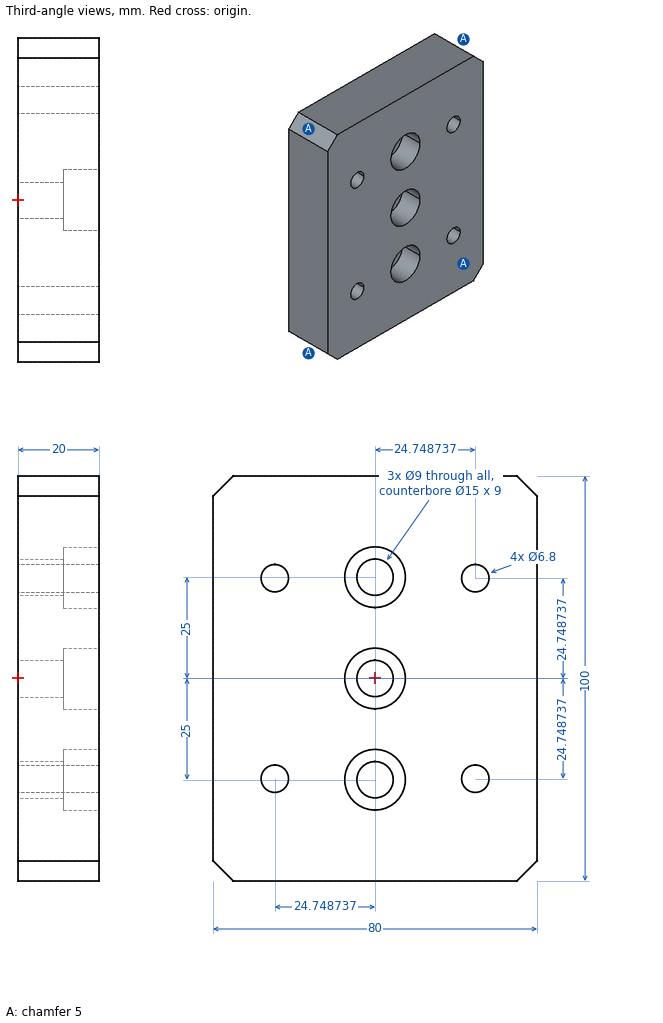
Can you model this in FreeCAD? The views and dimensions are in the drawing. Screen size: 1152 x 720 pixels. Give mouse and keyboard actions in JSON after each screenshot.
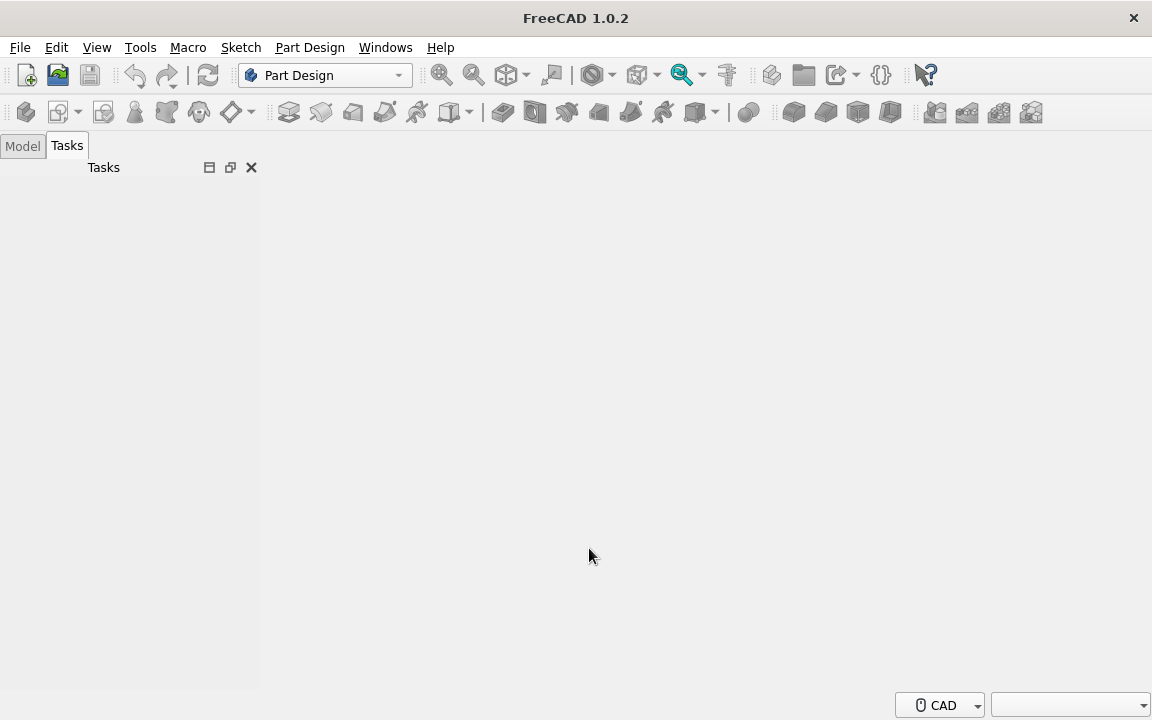
{"action": "key", "text": "ctrl+n"}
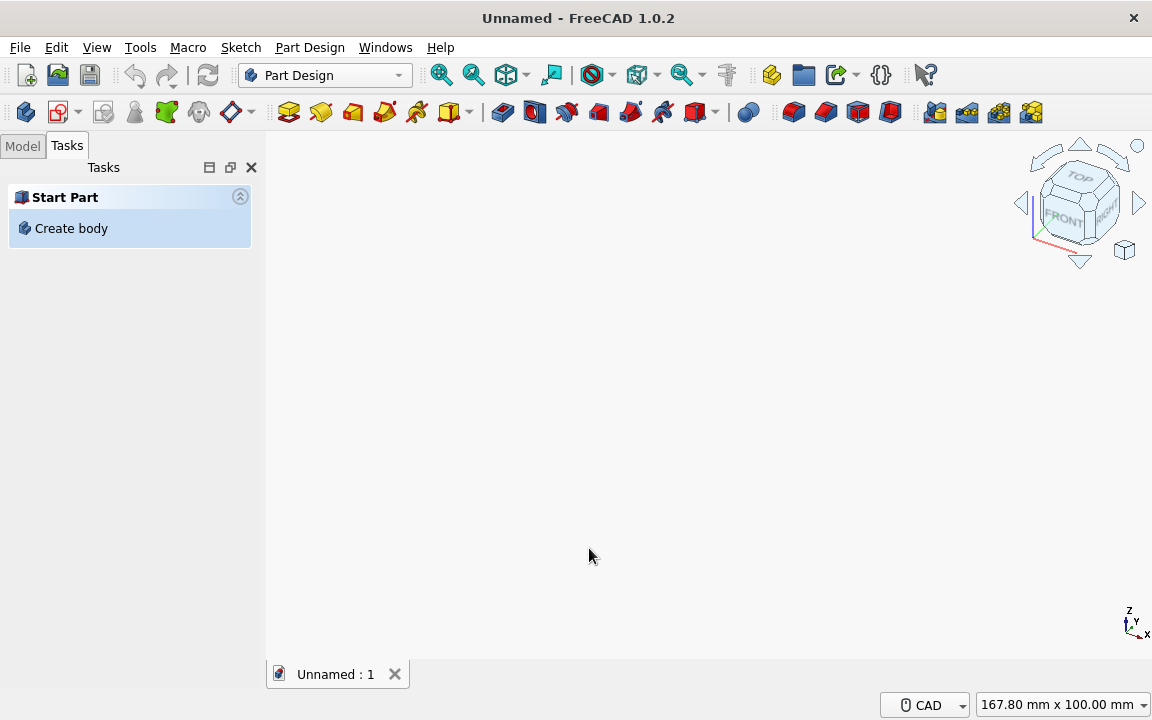
{"action": "left_click", "coordinate": [58, 112]}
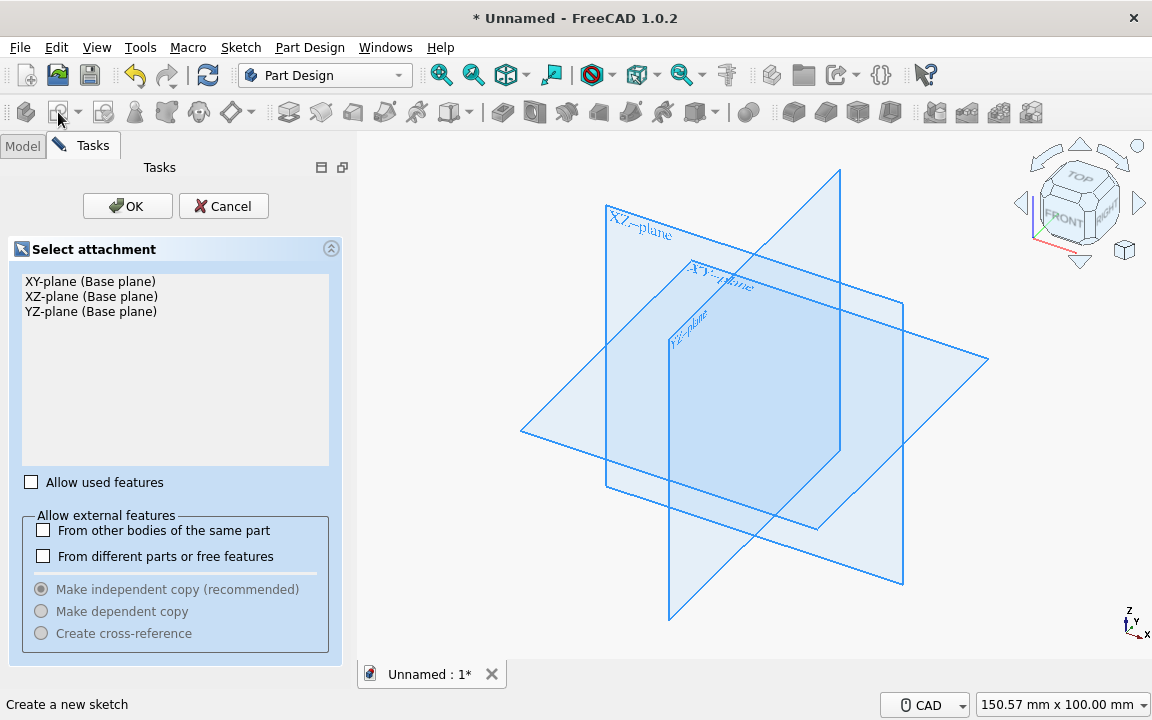
{"action": "left_click", "coordinate": [82, 312]}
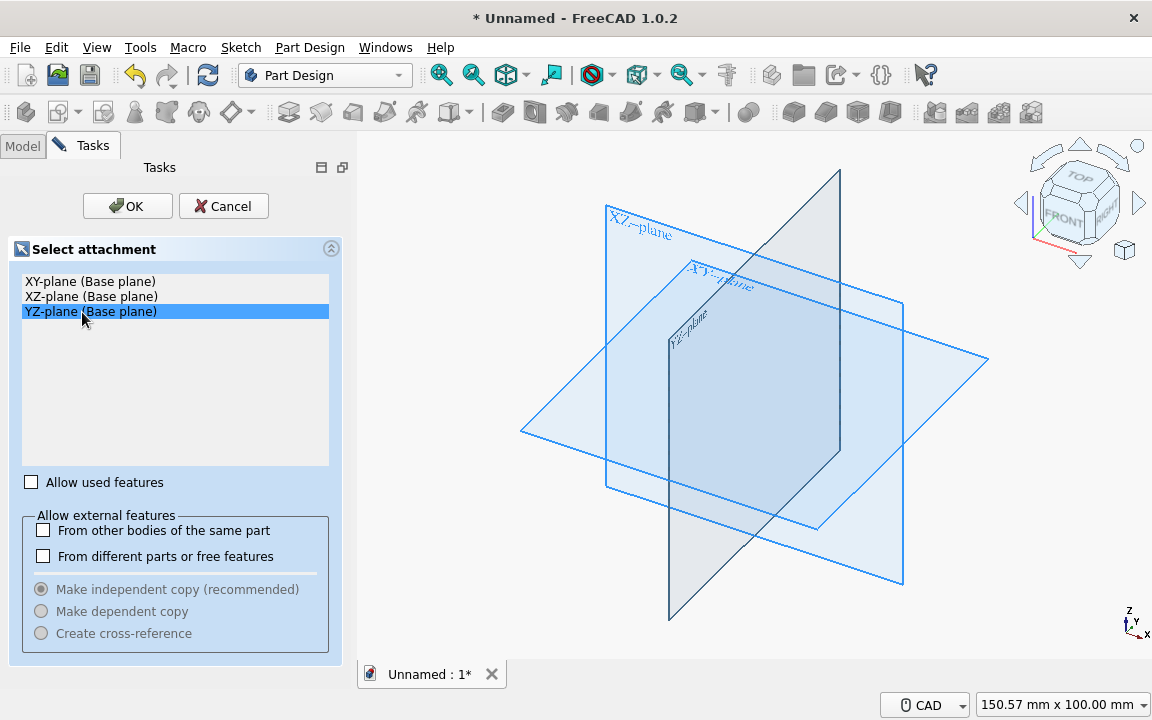
{"action": "left_click", "coordinate": [128, 206]}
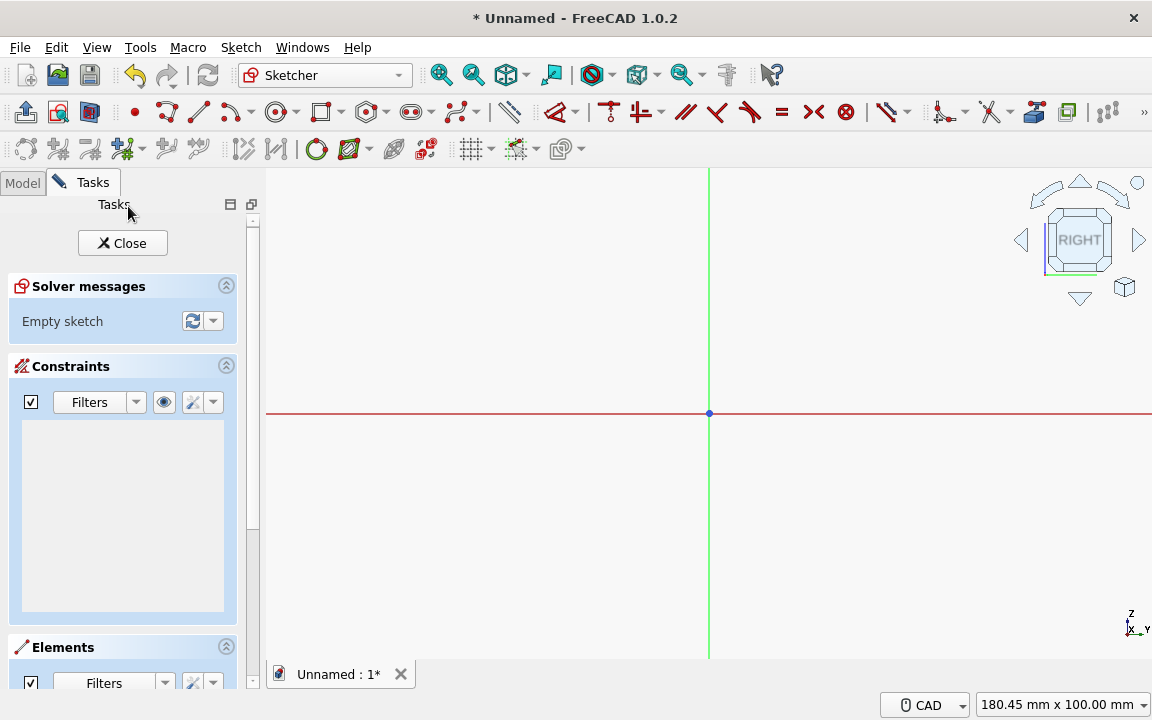
{"action": "scroll", "coordinate": [501, 414], "scroll_direction": "down", "scroll_amount": 2}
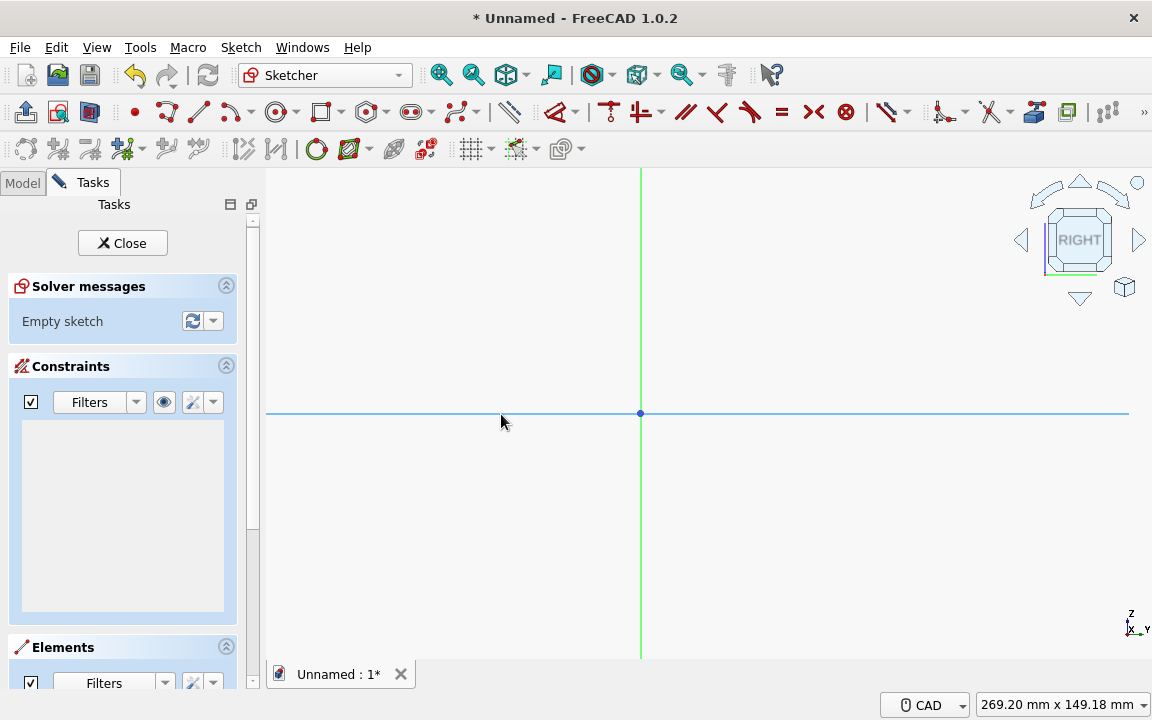
{"action": "key", "text": "g v"}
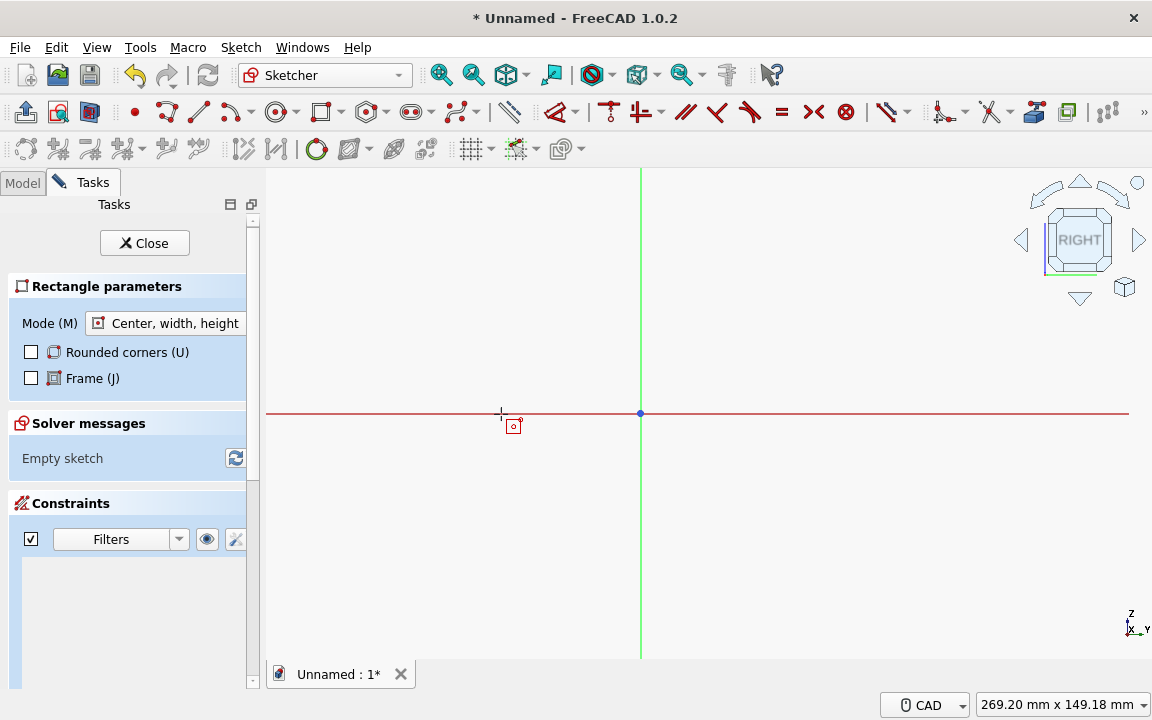
{"action": "left_click", "coordinate": [641, 414]}
{"action": "mouse_move", "coordinate": [772, 249]}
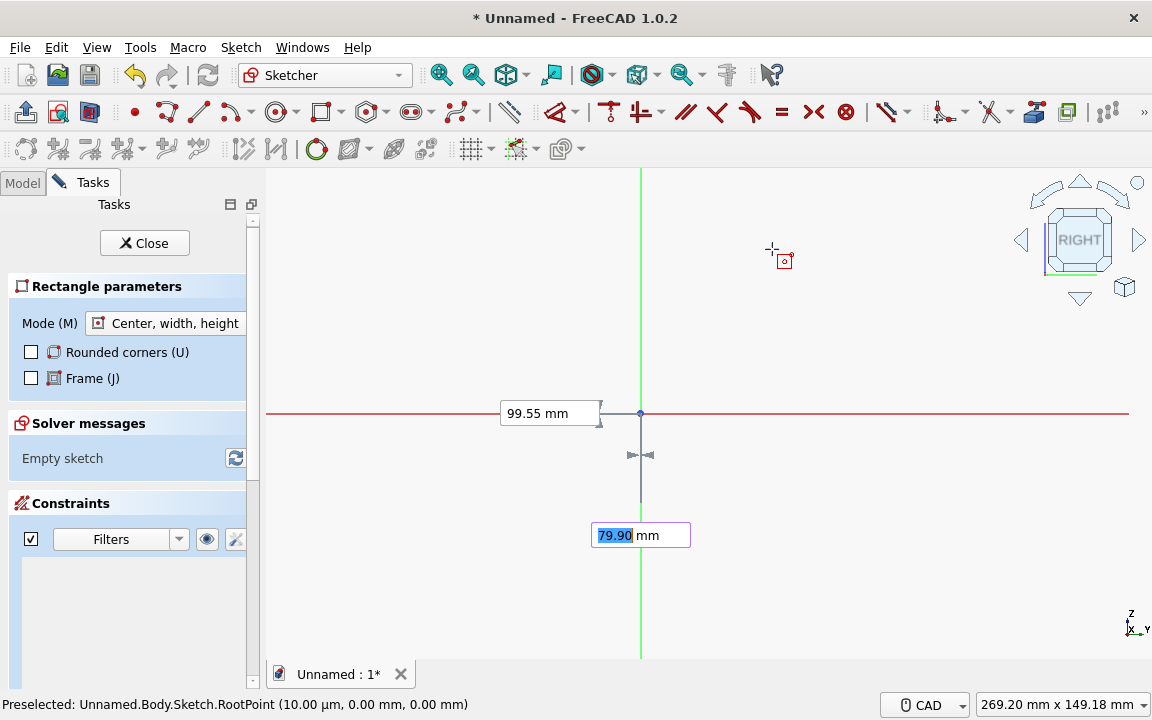
{"action": "type", "text": "80"}
{"action": "key", "text": "Tab"}
{"action": "type", "text": "100"}
{"action": "key", "text": "Return"}
{"action": "key", "text": "Escape"}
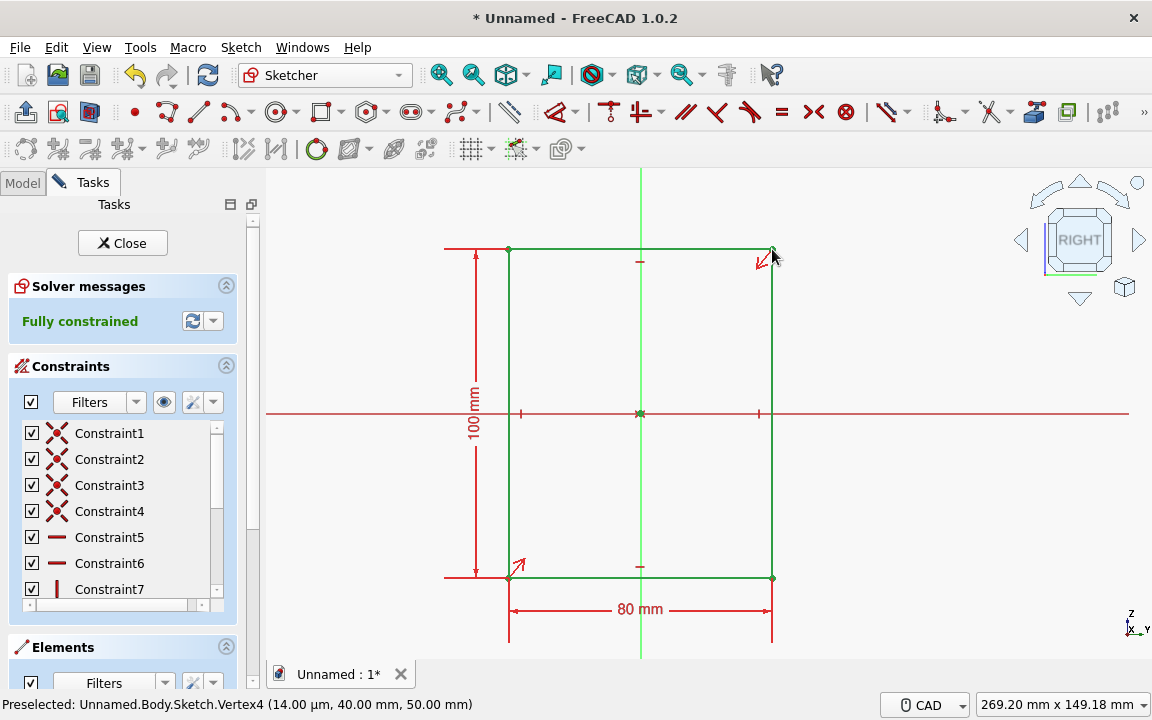
{"action": "left_click", "coordinate": [123, 243]}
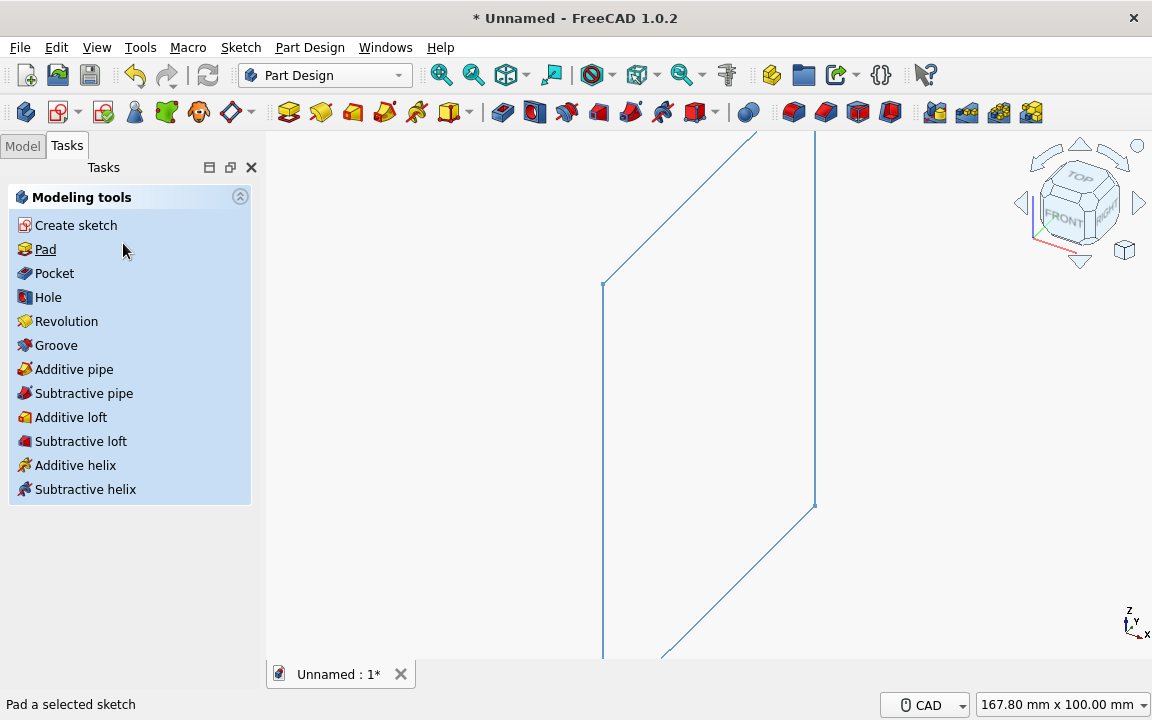
{"action": "left_click", "coordinate": [290, 112]}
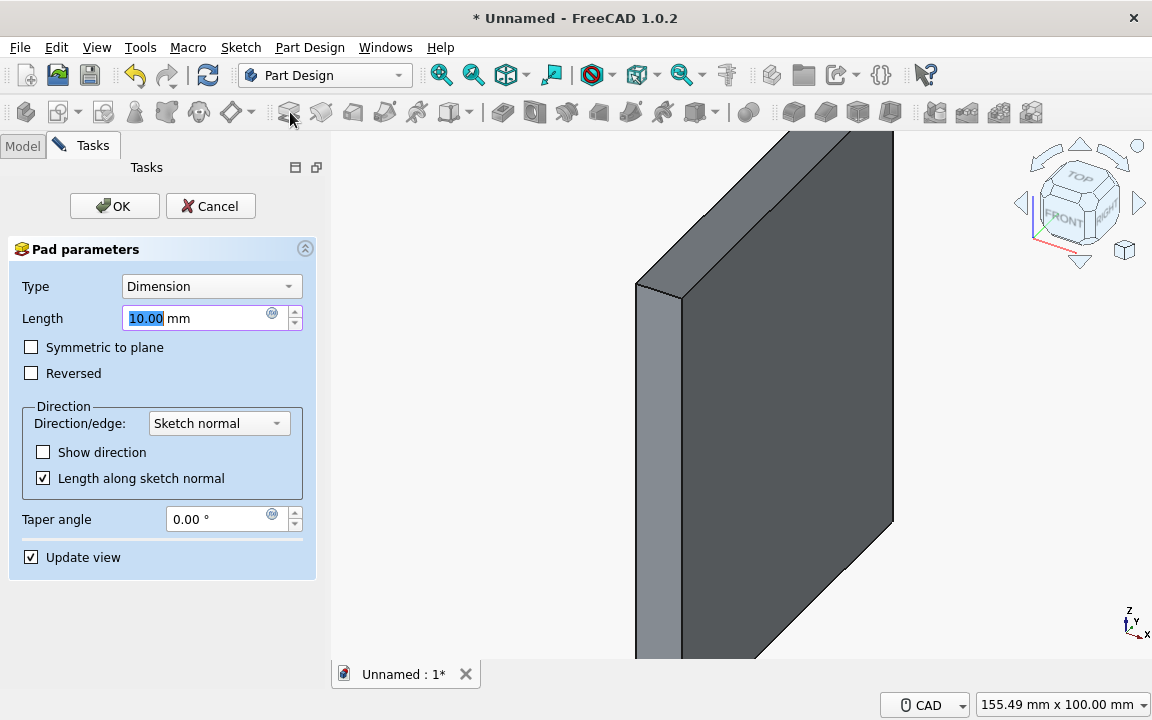
{"action": "type", "text": "20"}
{"action": "key", "text": "Tab"}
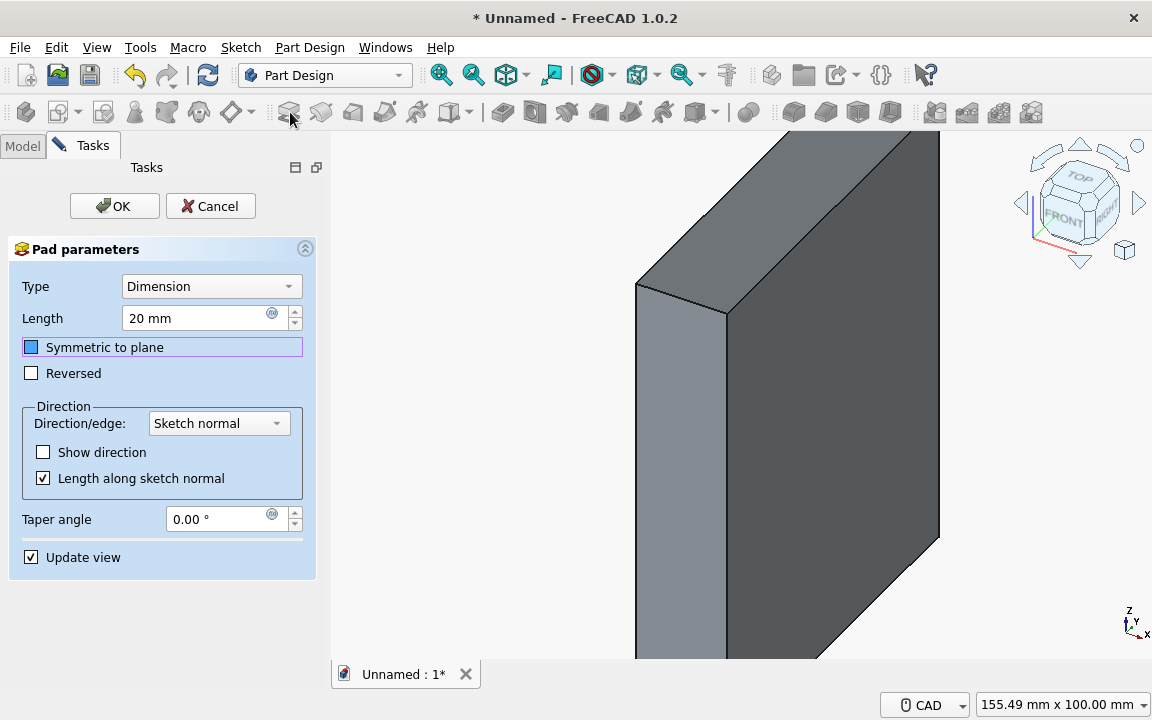
{"action": "left_click", "coordinate": [115, 206]}